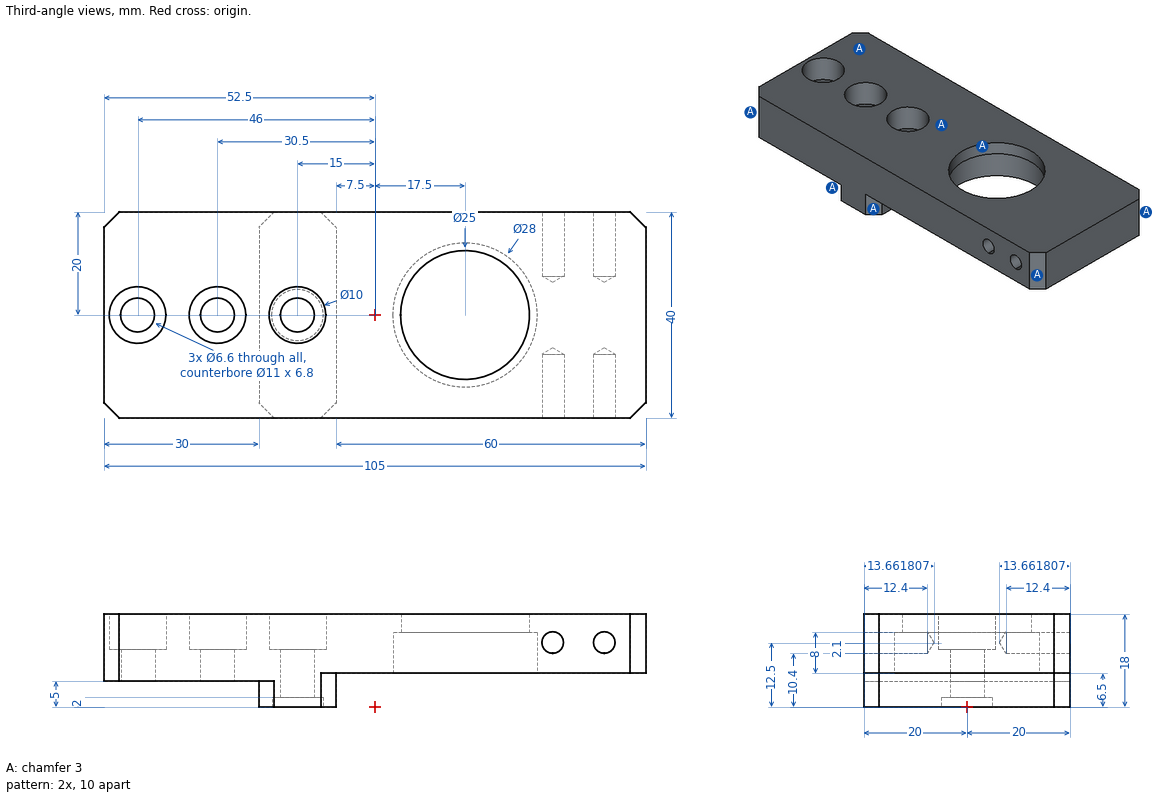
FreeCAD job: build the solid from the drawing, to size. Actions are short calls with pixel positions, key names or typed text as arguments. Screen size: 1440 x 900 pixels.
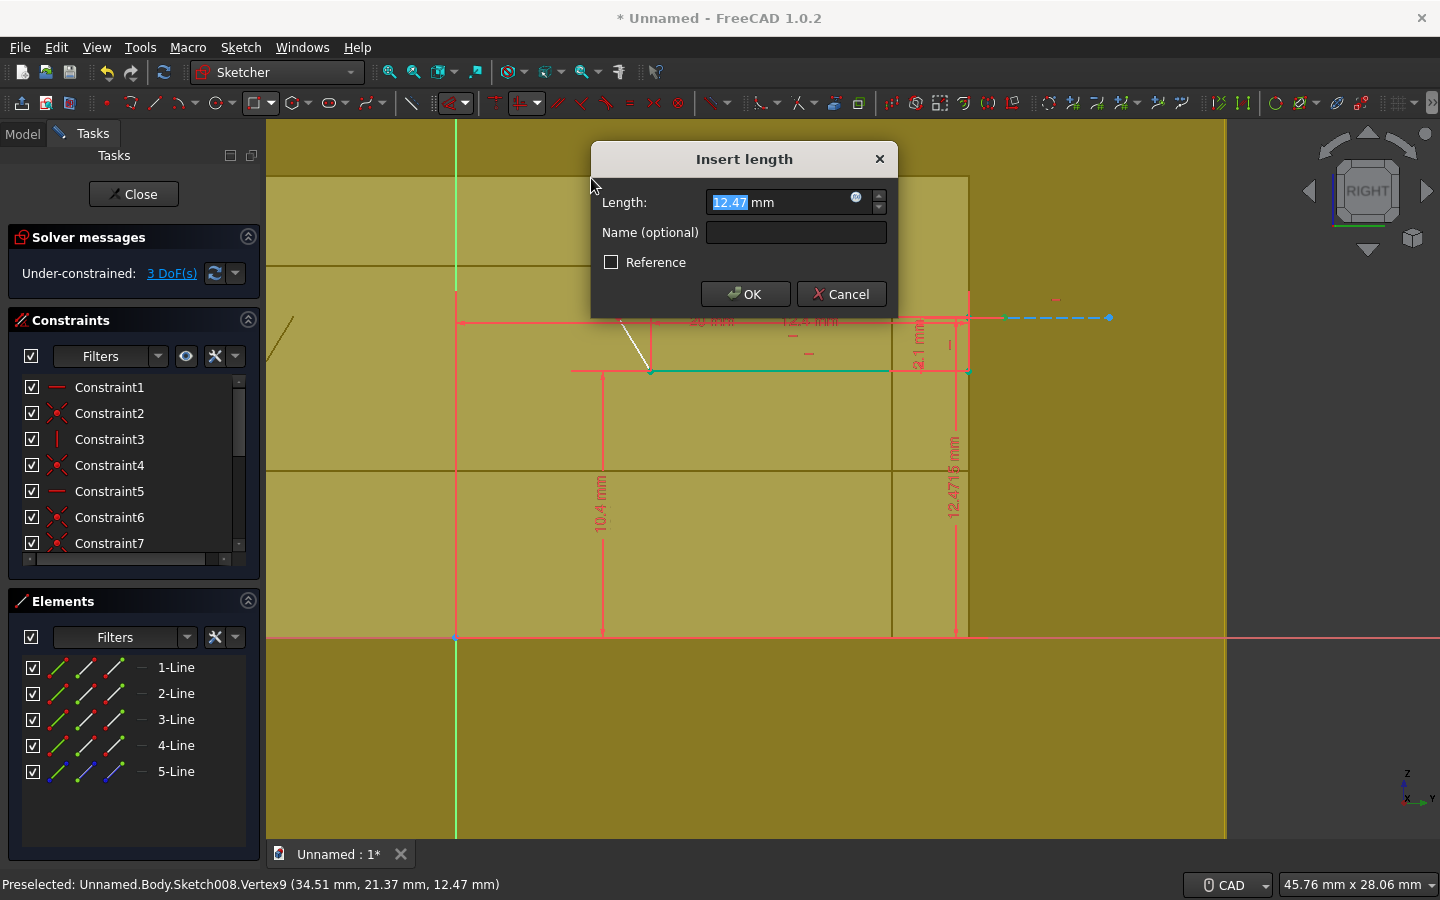
text(12.5)
key(Return)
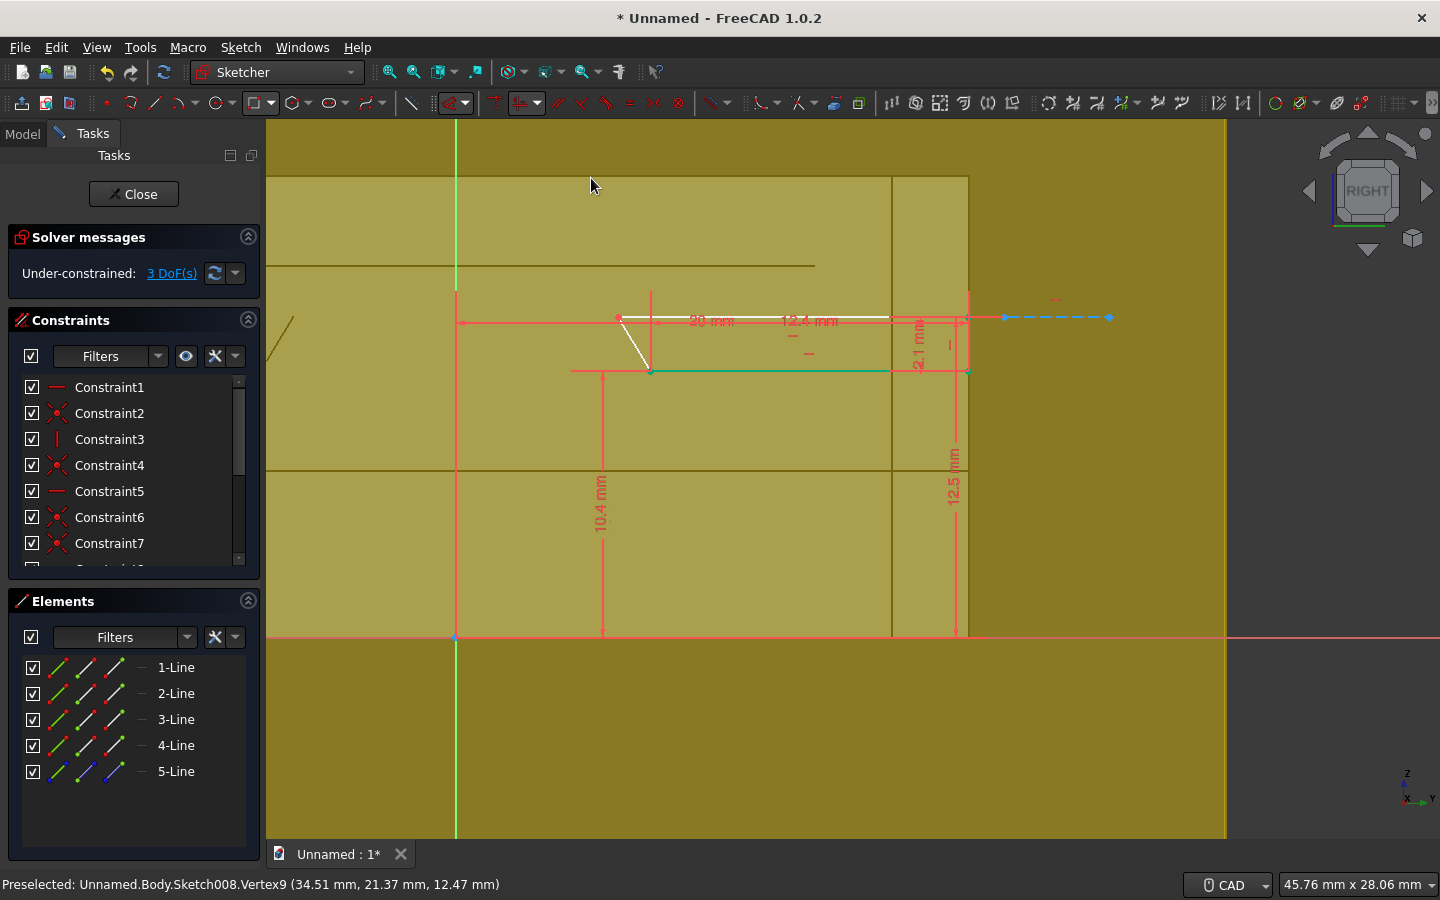
click(864, 317)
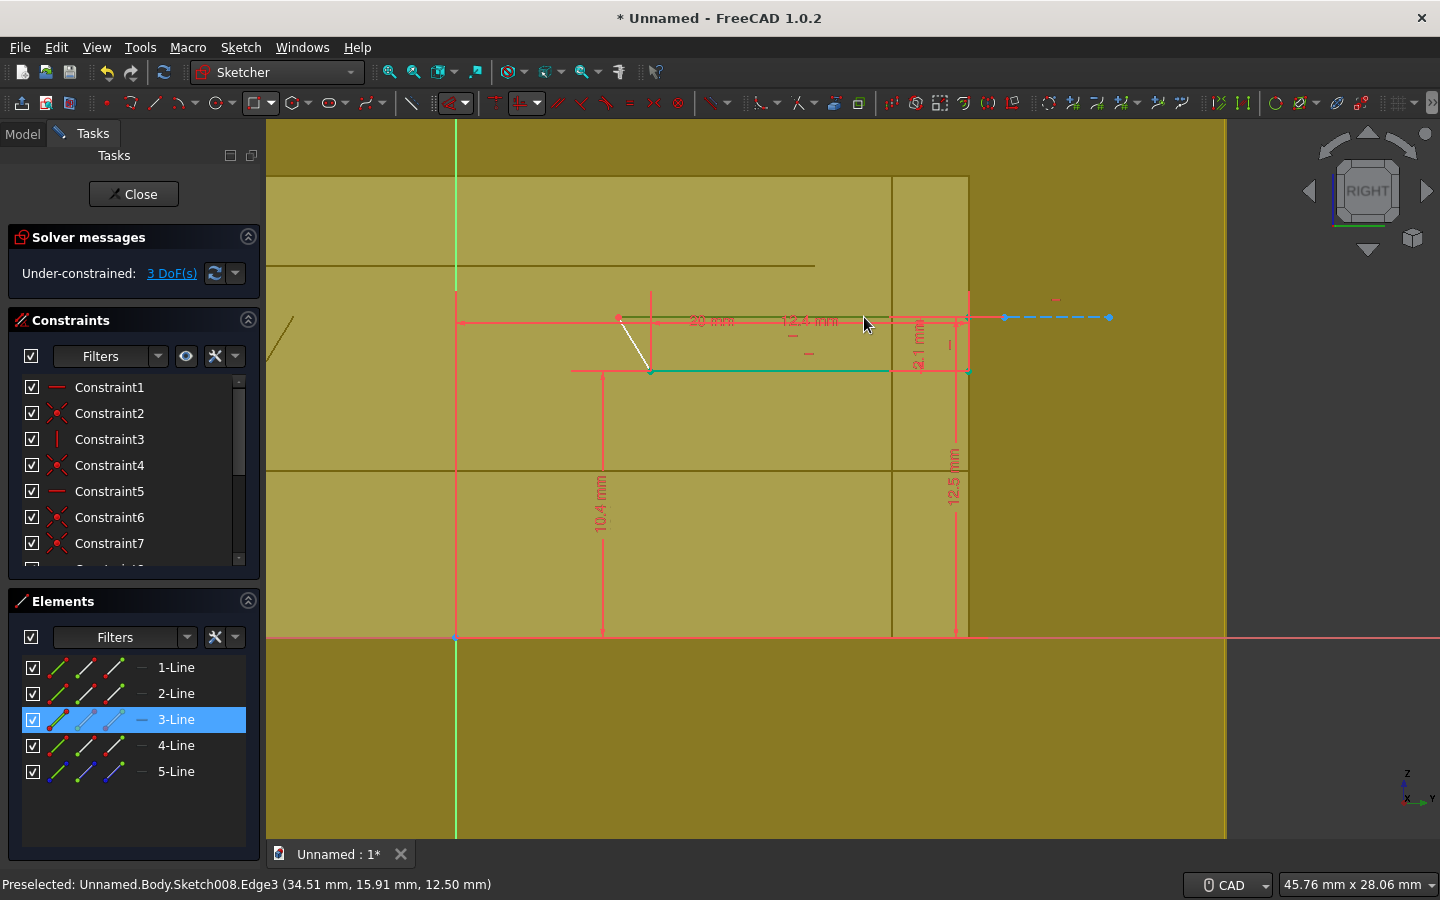
key(l)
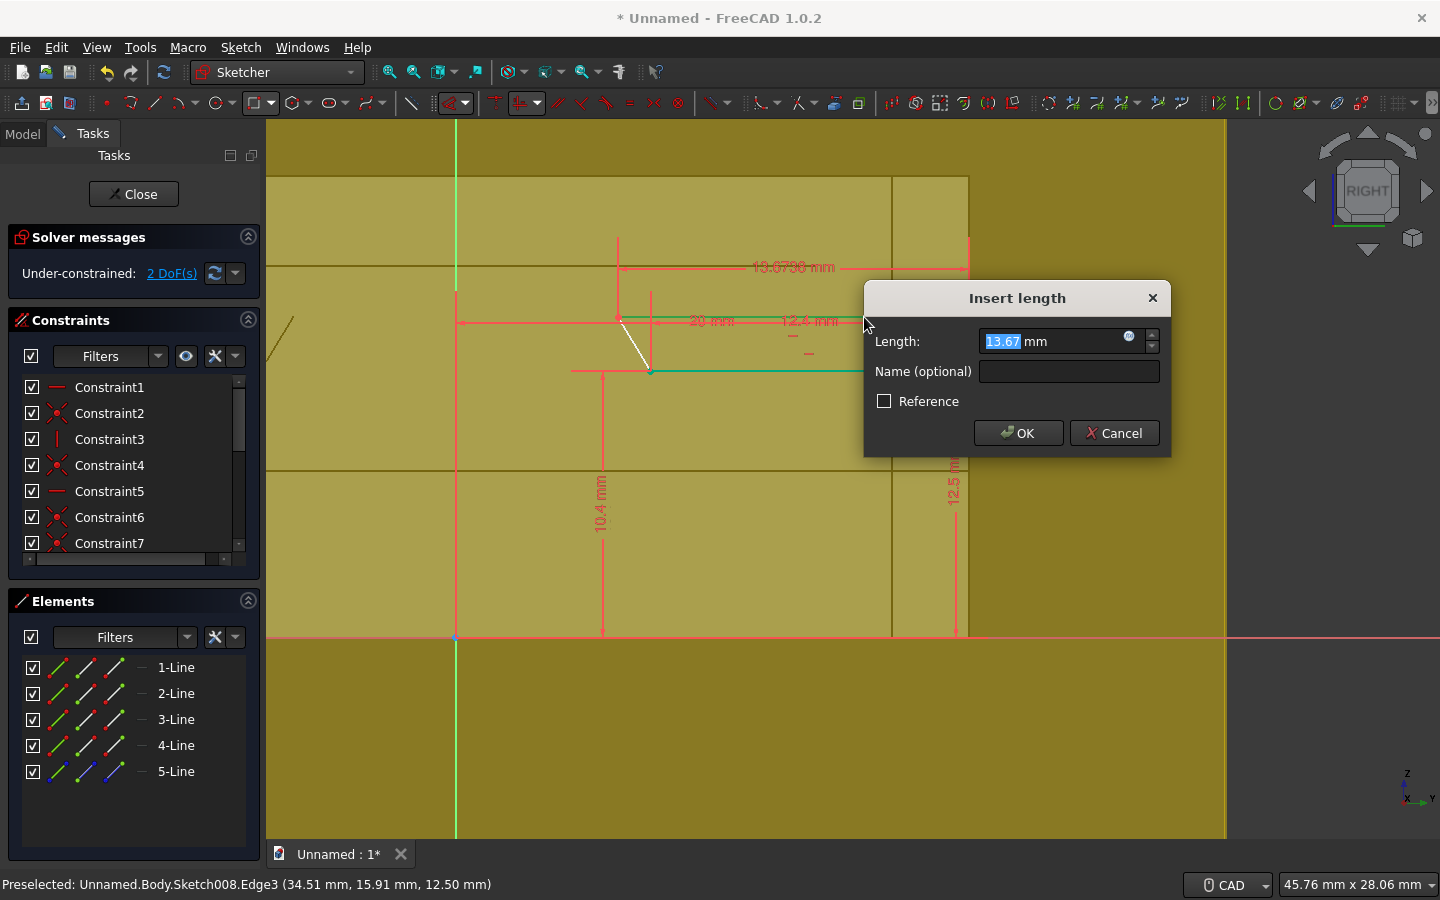
text(13.661807)
key(Return)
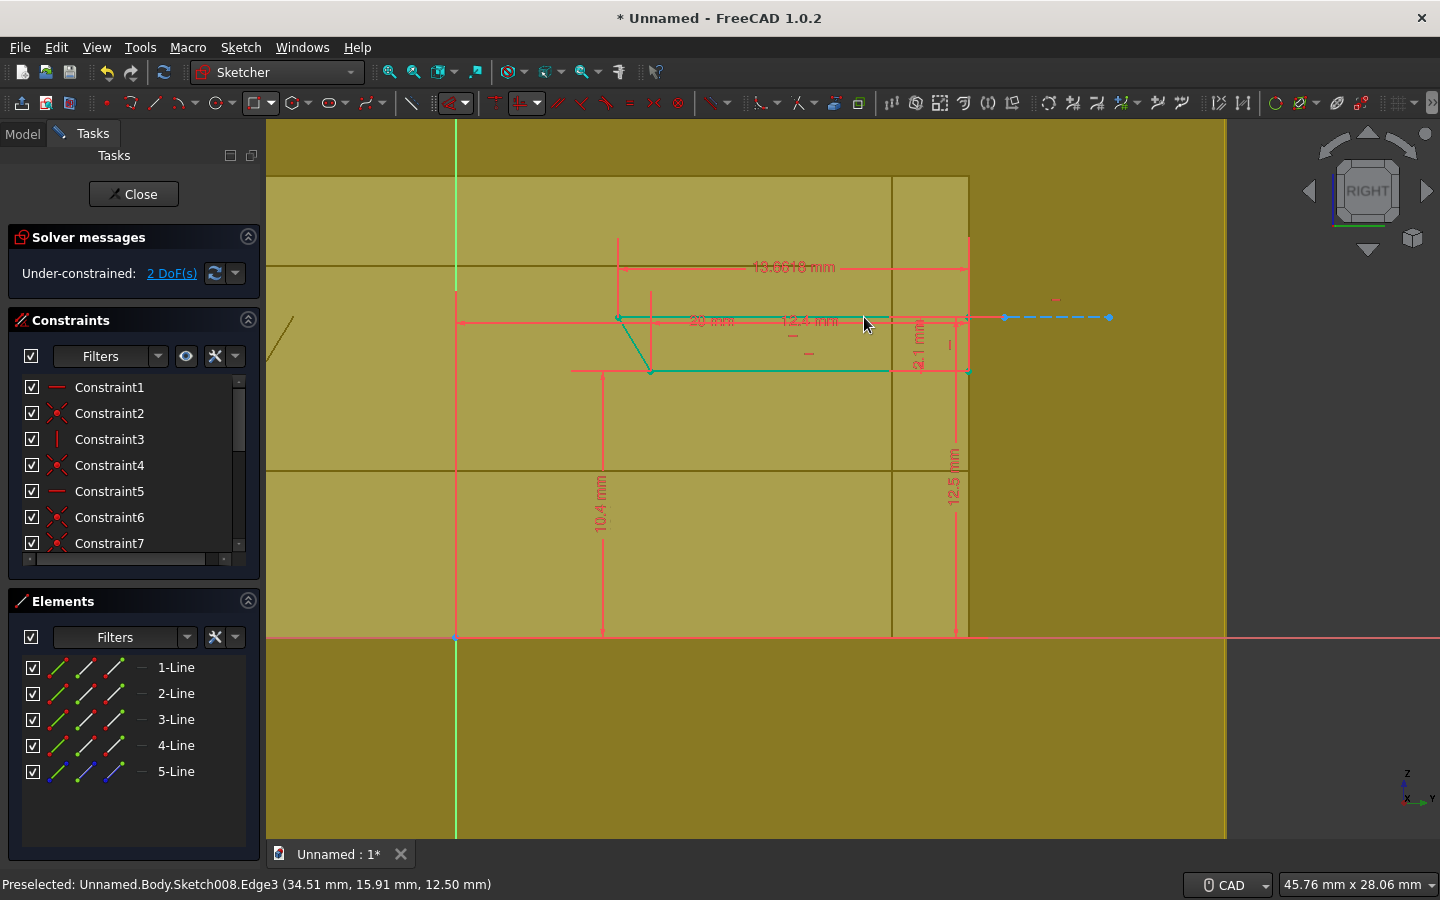
click(134, 194)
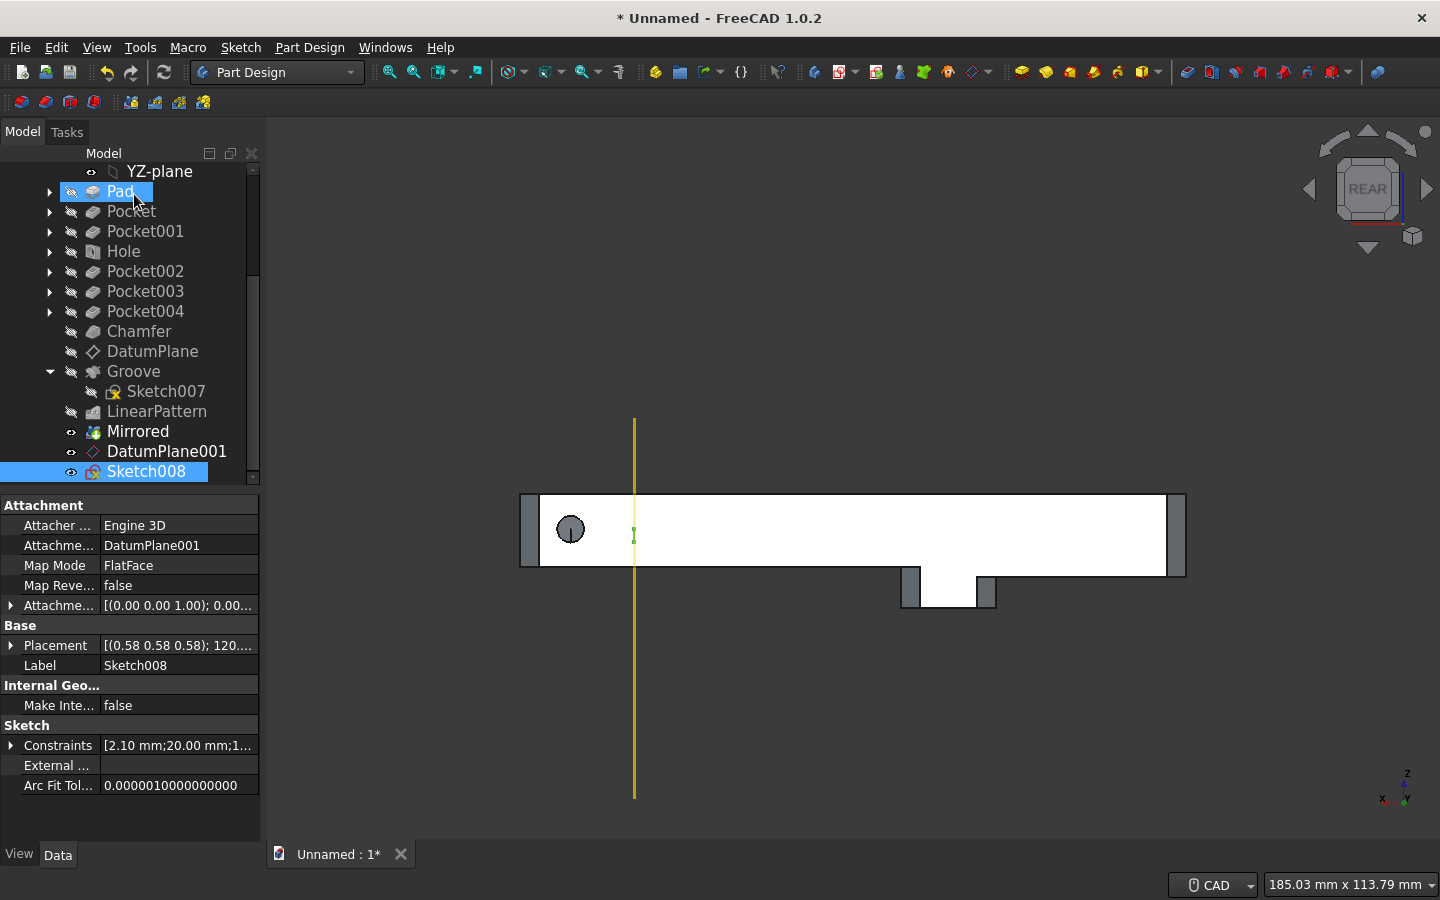
click(1236, 72)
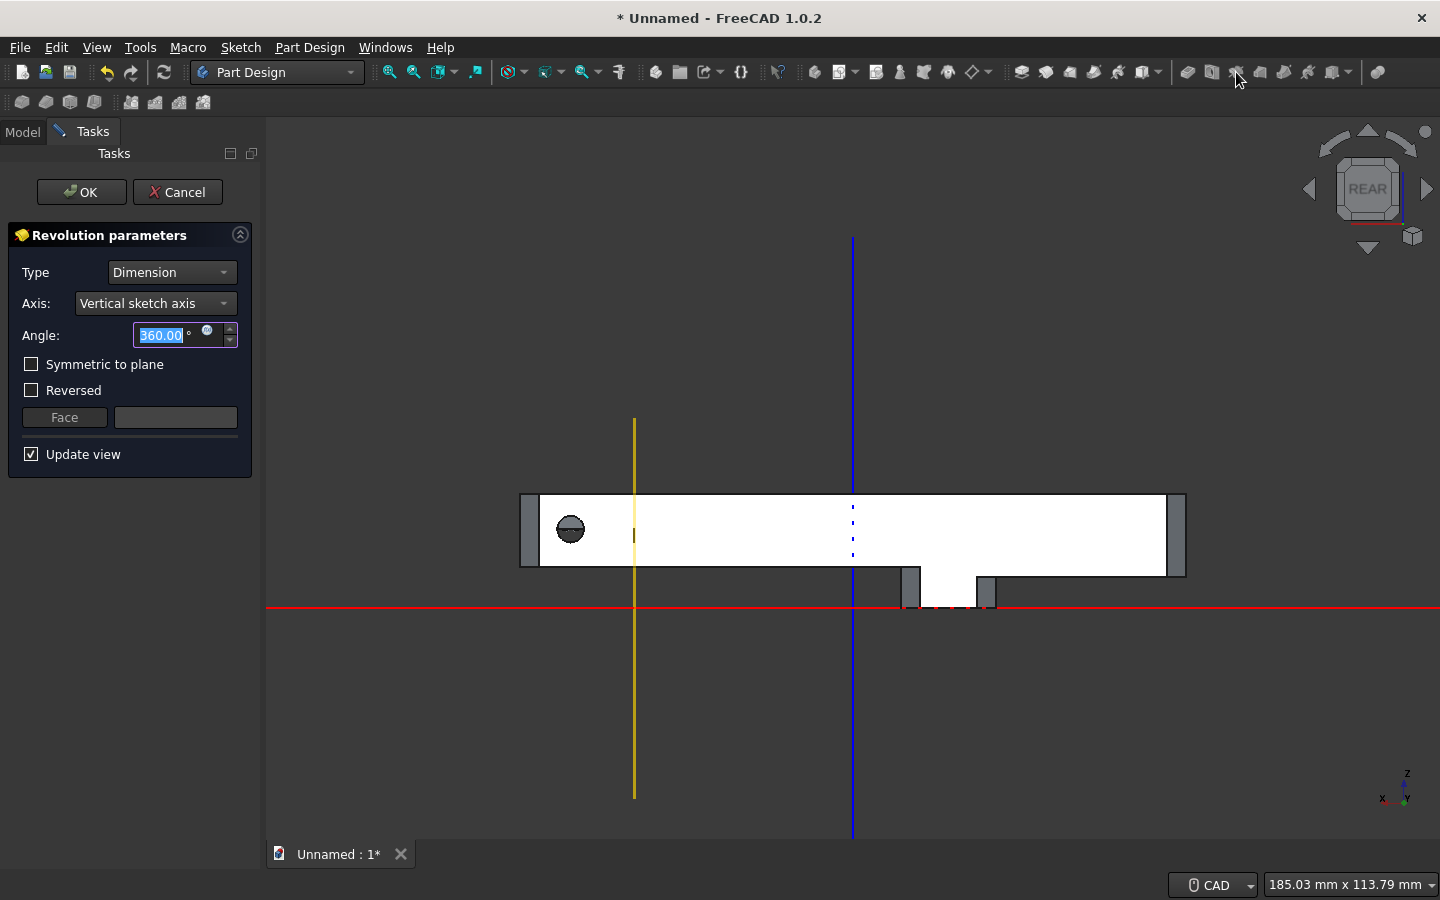
click(156, 304)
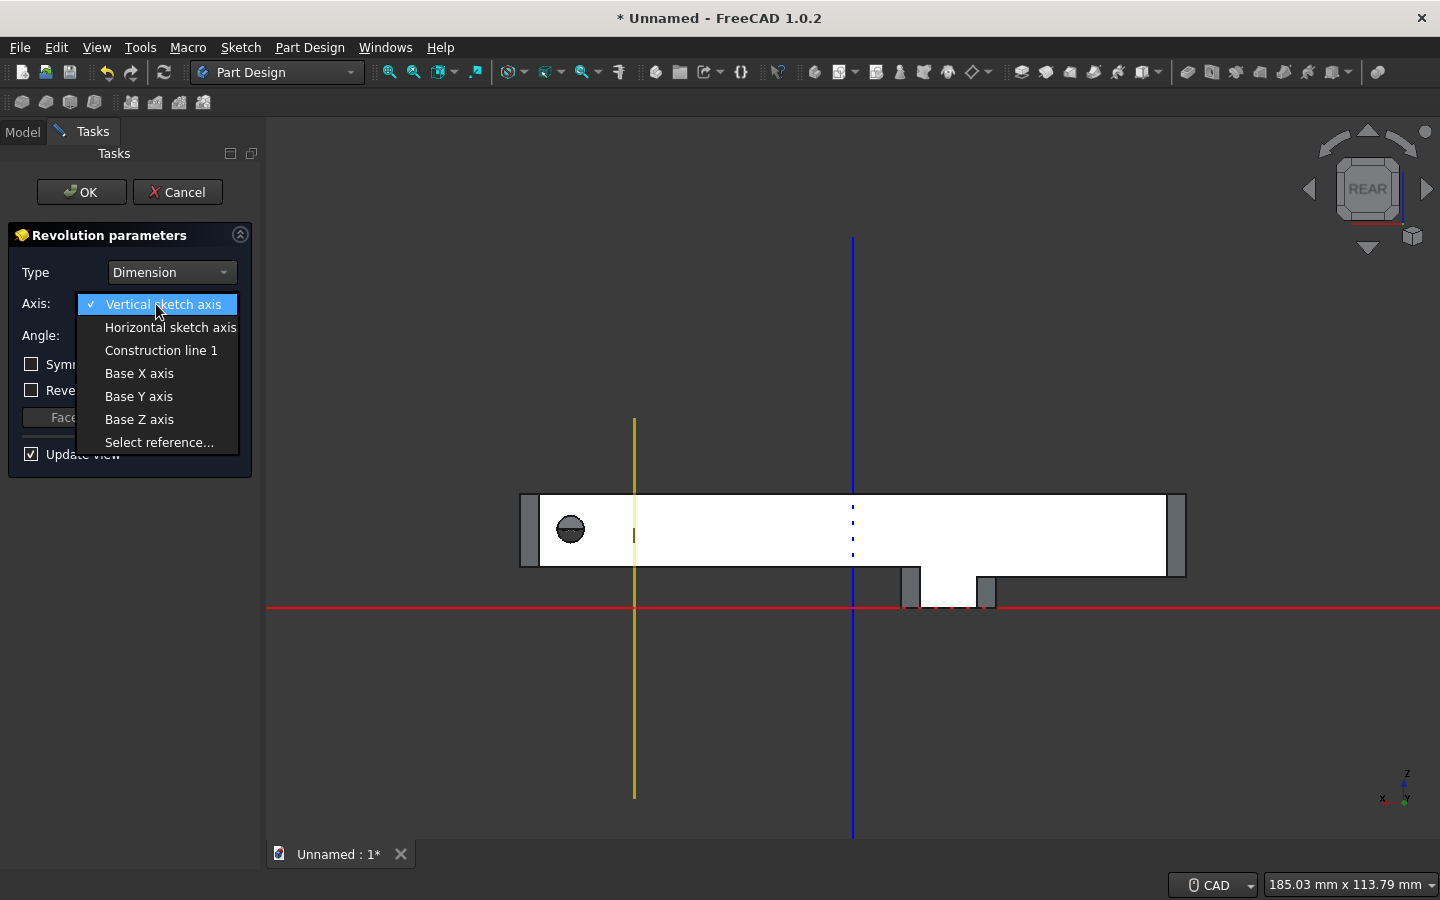
click(156, 350)